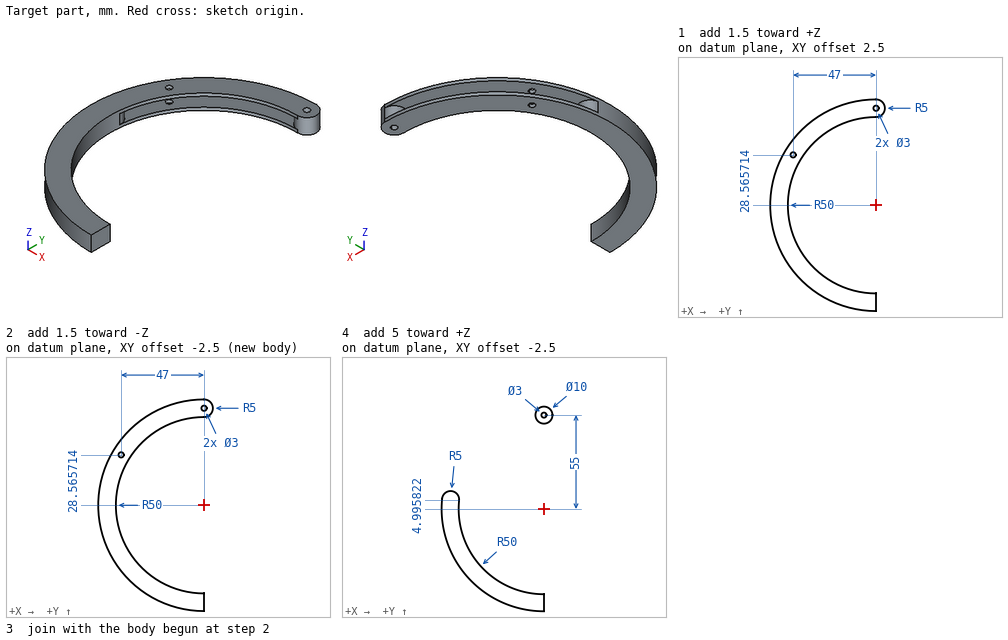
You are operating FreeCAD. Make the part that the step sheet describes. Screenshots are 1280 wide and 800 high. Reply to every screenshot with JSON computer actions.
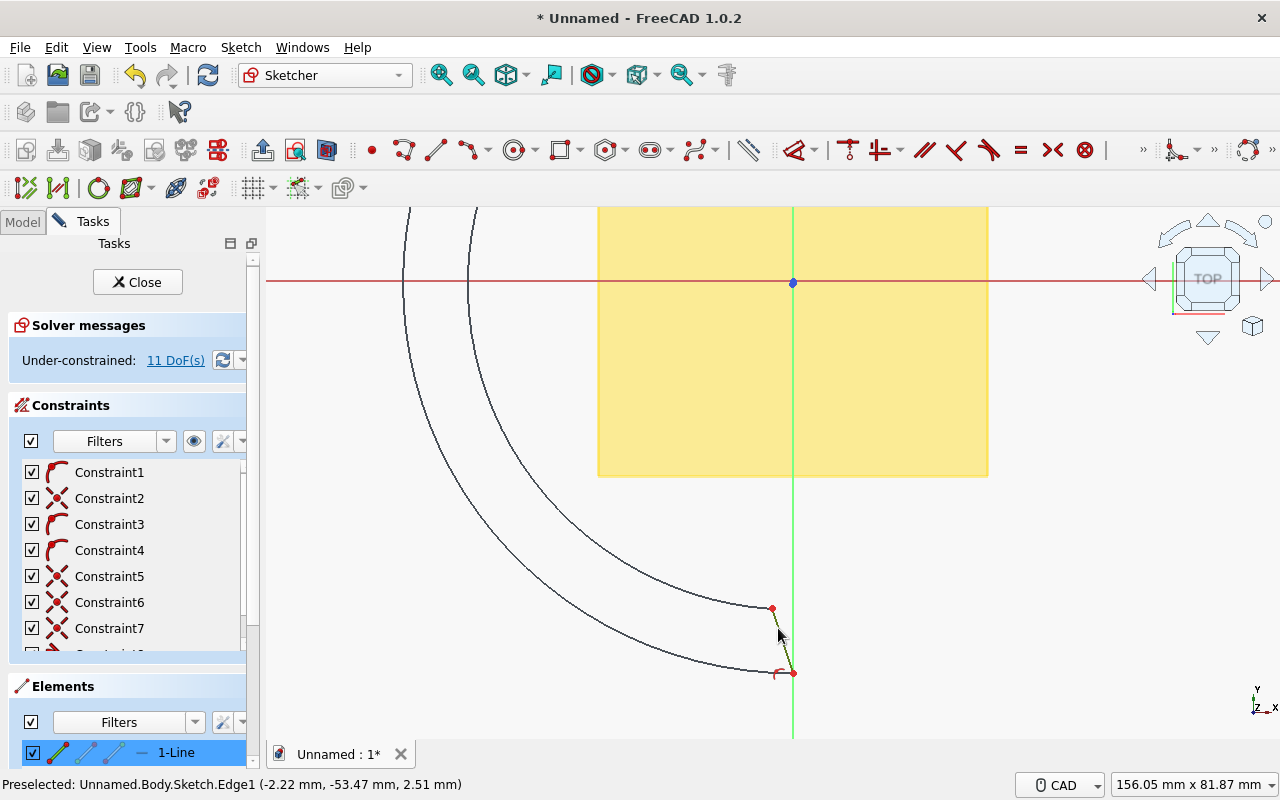
{"action": "key", "text": "v"}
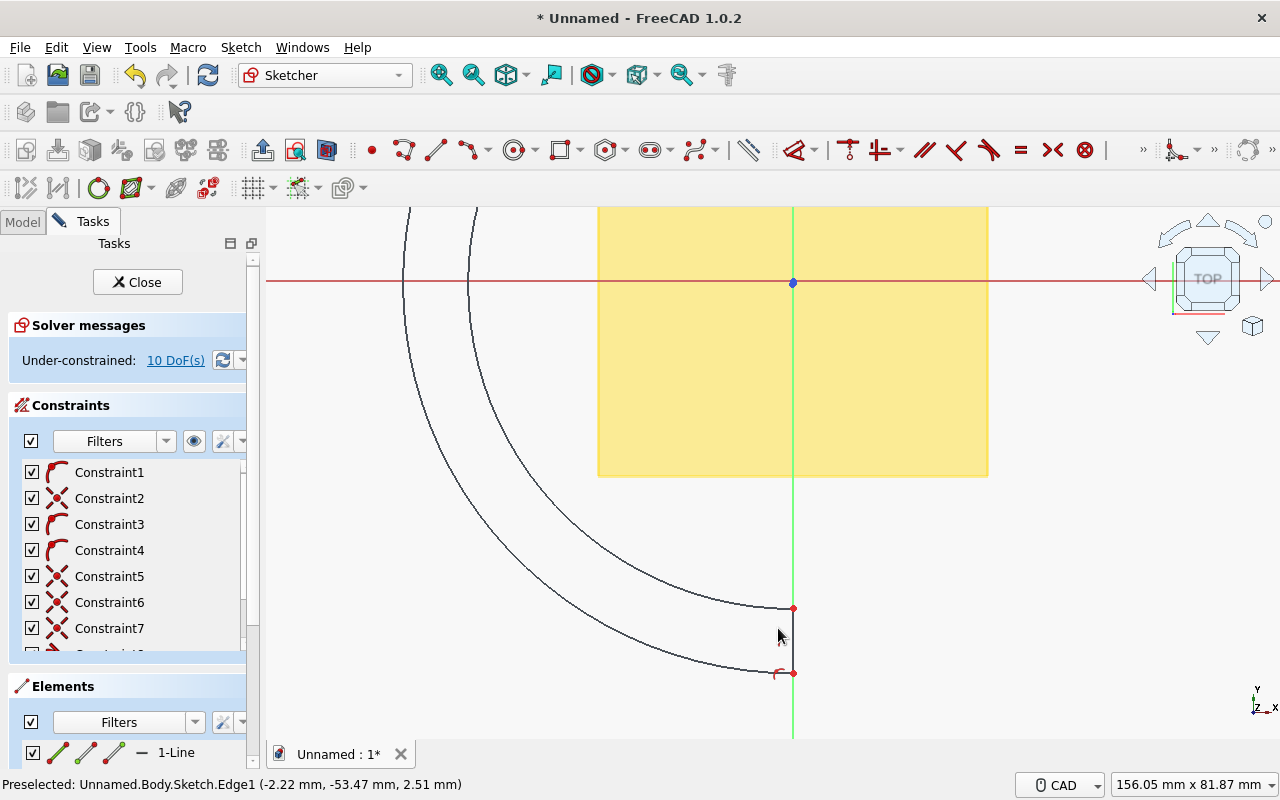
{"action": "left_click", "coordinate": [530, 475]}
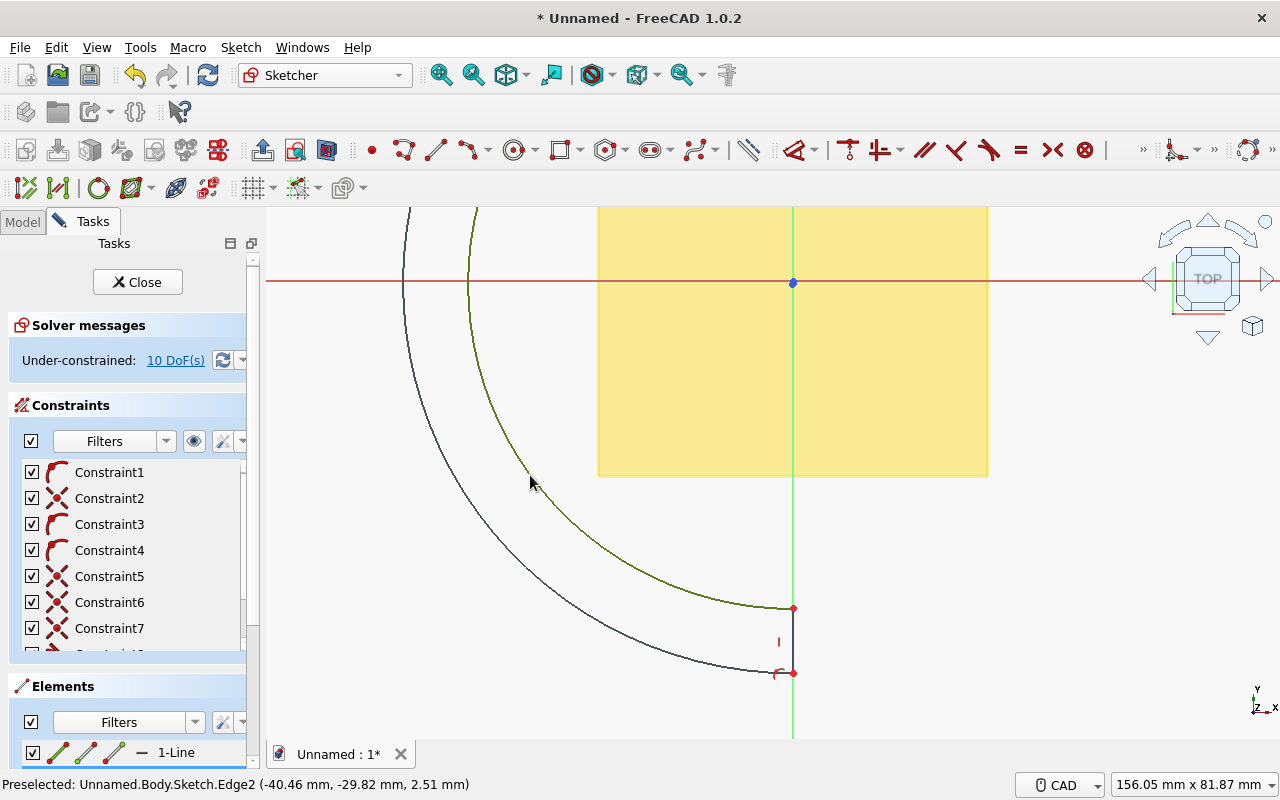
{"action": "left_click", "coordinate": [478, 512]}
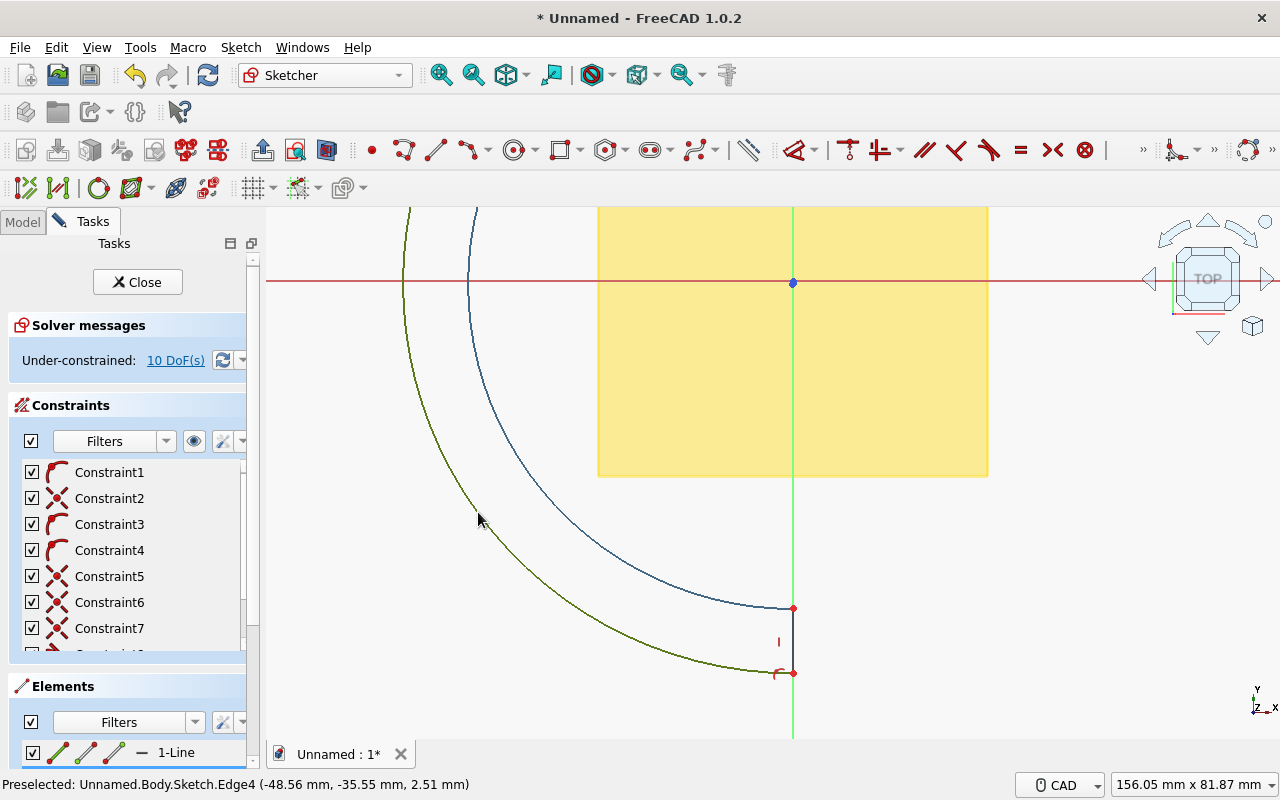
{"action": "left_click", "coordinate": [848, 150]}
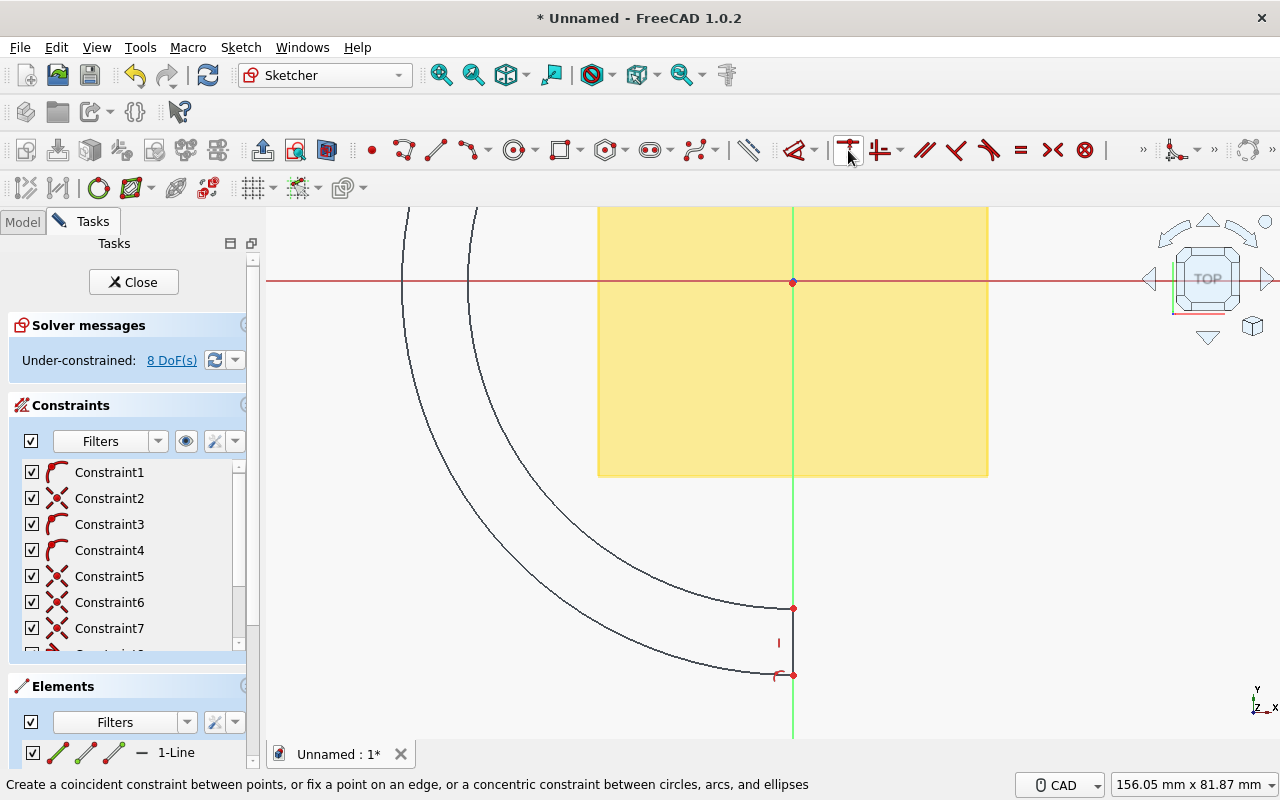
{"action": "scroll", "coordinate": [793, 283], "scroll_direction": "up", "scroll_amount": 9}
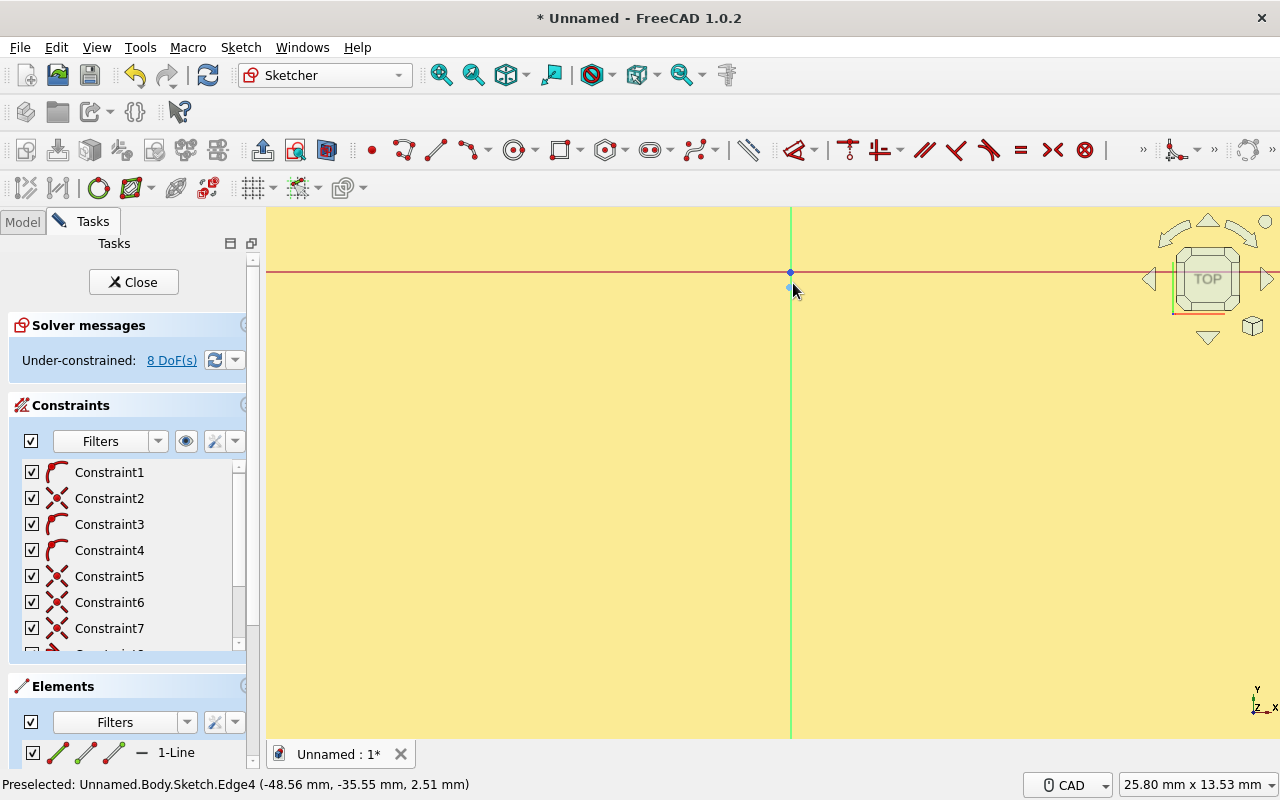
{"action": "left_click_drag", "start_coordinate": [780, 262], "coordinate": [801, 298]}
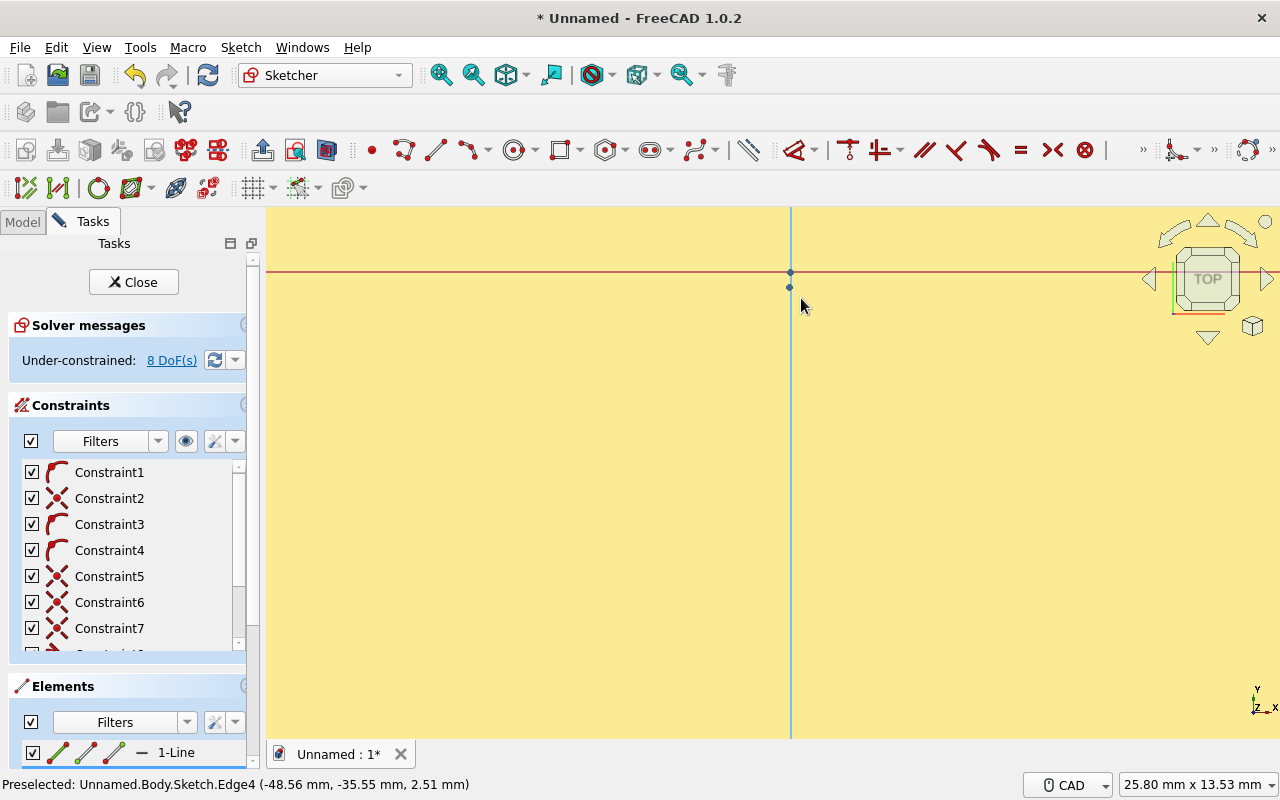
{"action": "left_click", "coordinate": [848, 150]}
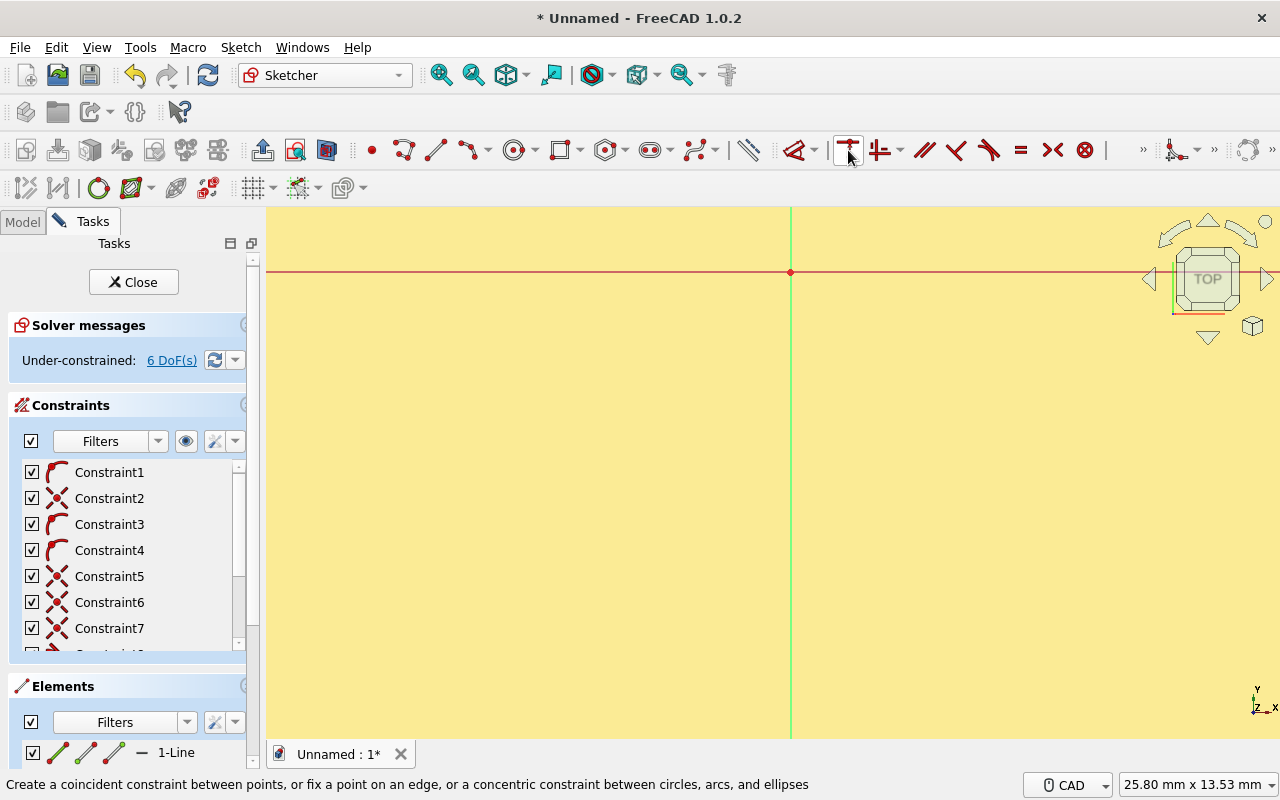
{"action": "scroll", "coordinate": [784, 489], "scroll_direction": "down", "scroll_amount": 13}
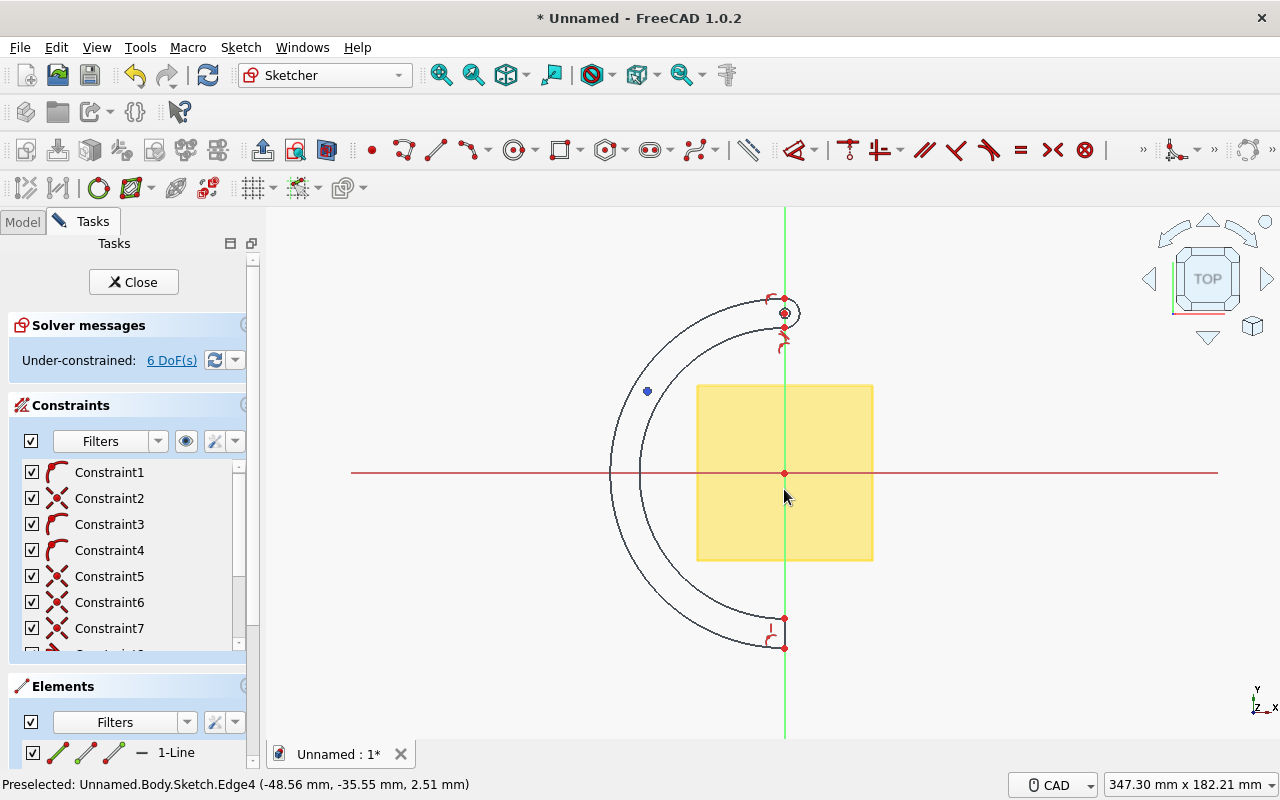
{"action": "scroll", "coordinate": [650, 389], "scroll_direction": "up", "scroll_amount": 7}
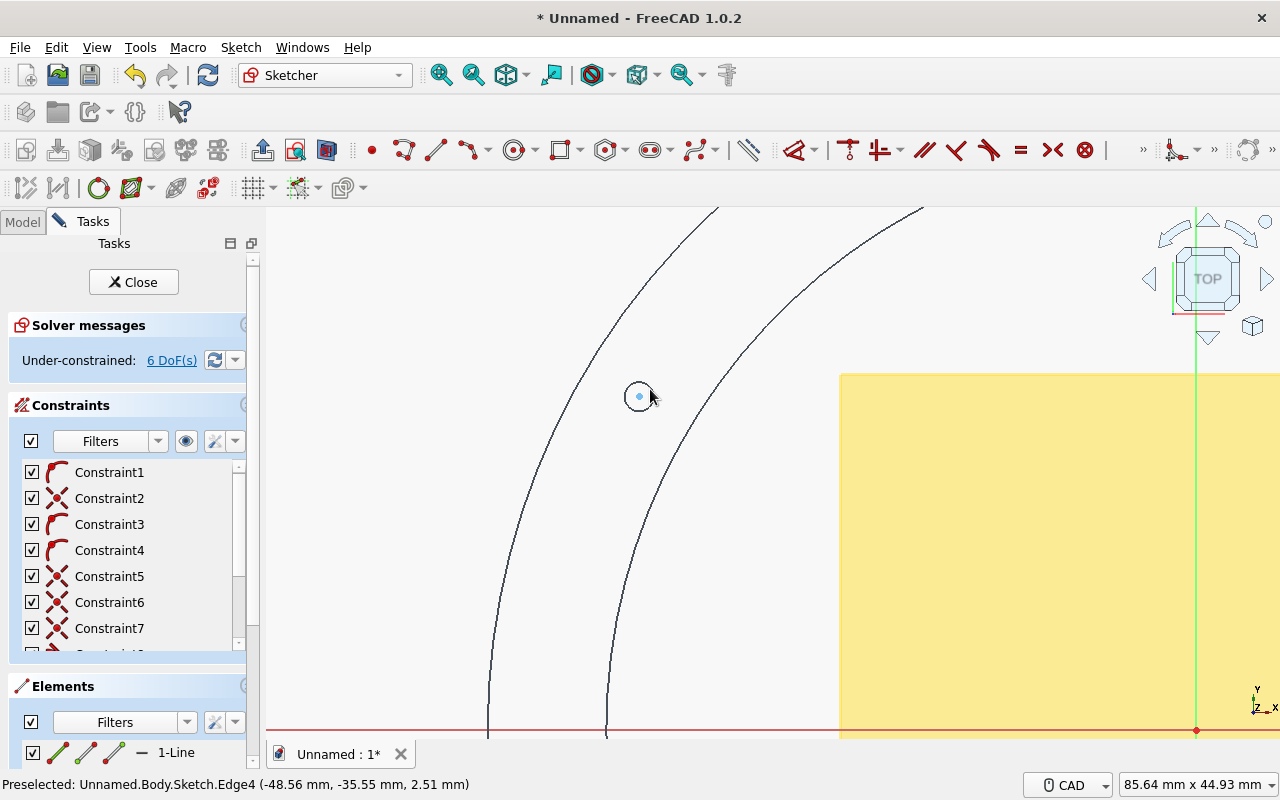
{"action": "left_click", "coordinate": [649, 386]}